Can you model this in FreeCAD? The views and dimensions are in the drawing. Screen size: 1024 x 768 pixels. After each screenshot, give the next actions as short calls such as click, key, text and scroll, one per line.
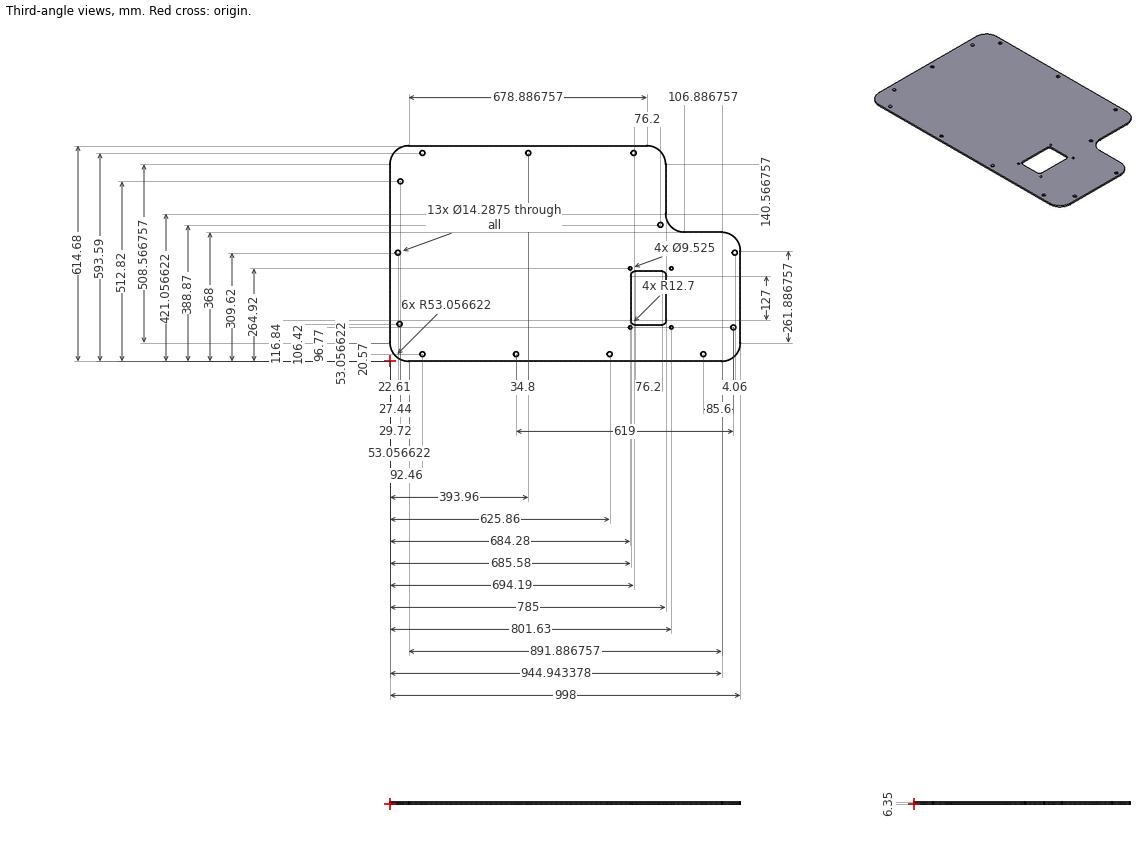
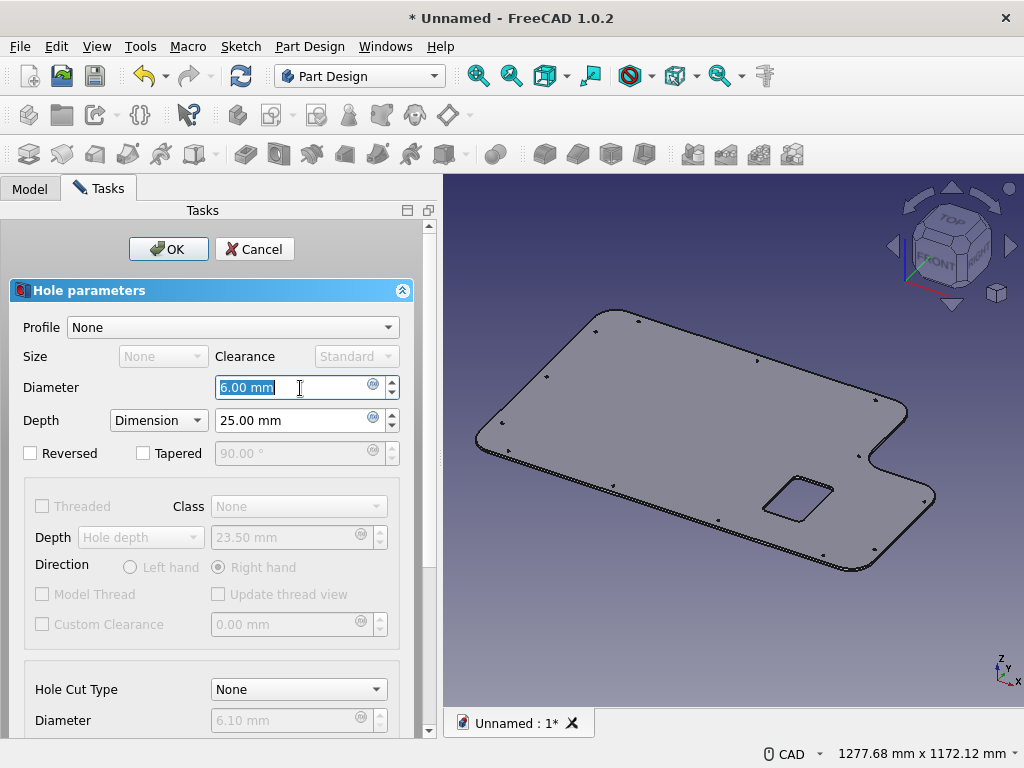
text(14.2875)
key(Tab)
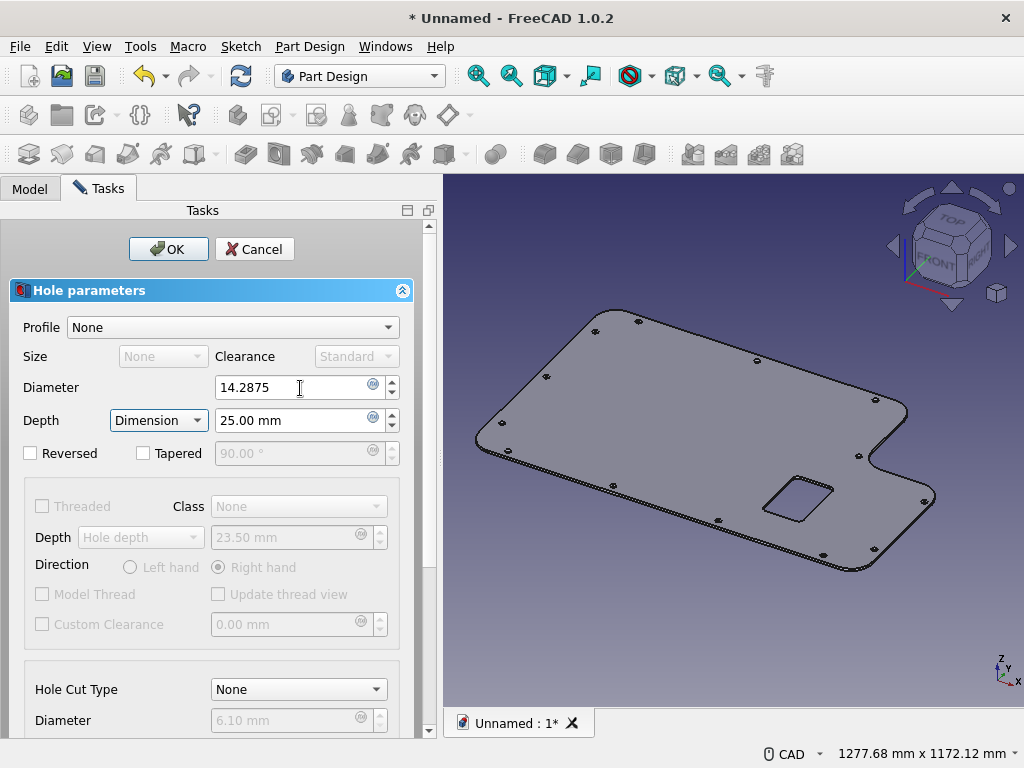
click(160, 420)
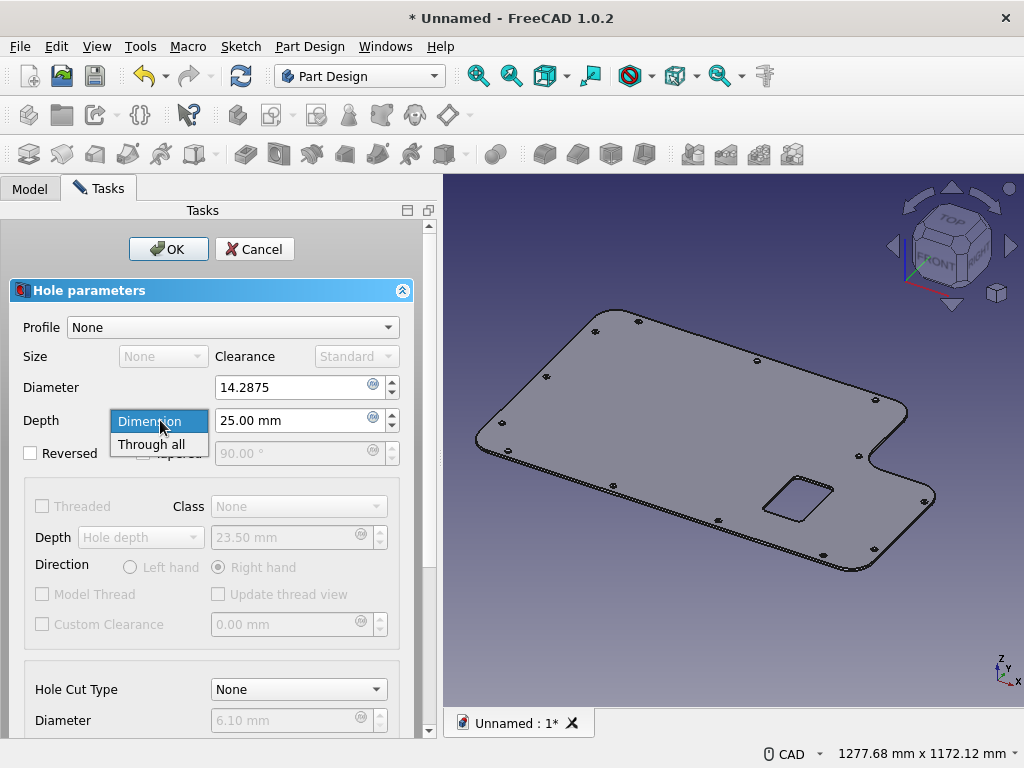
click(158, 444)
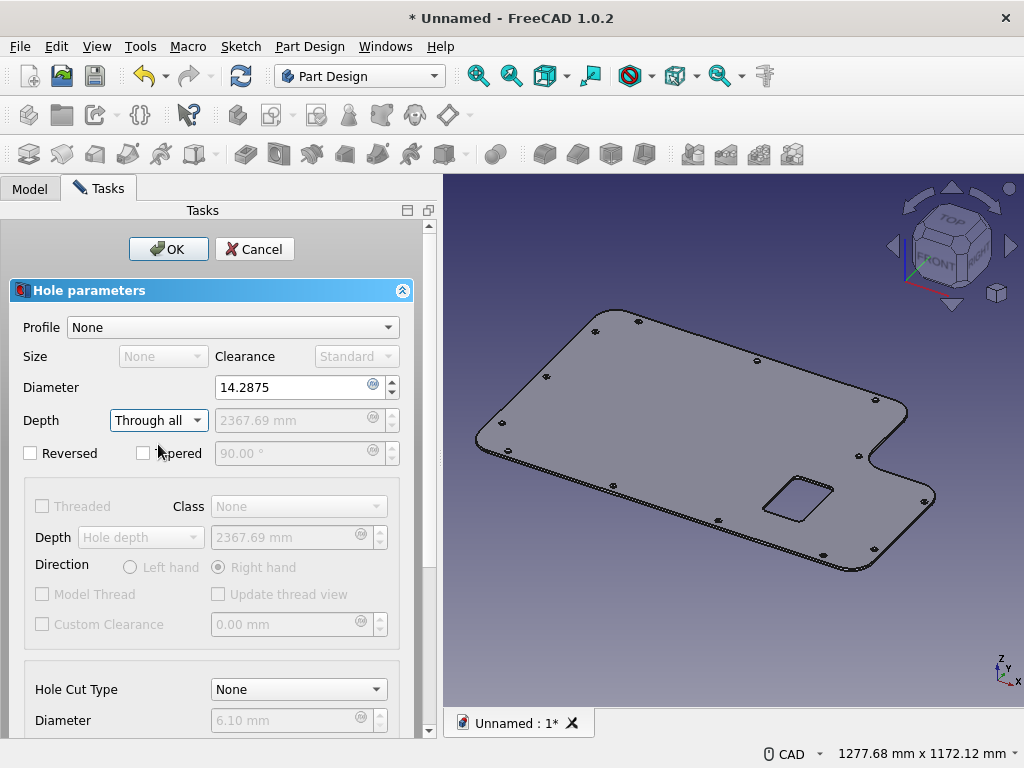
click(169, 249)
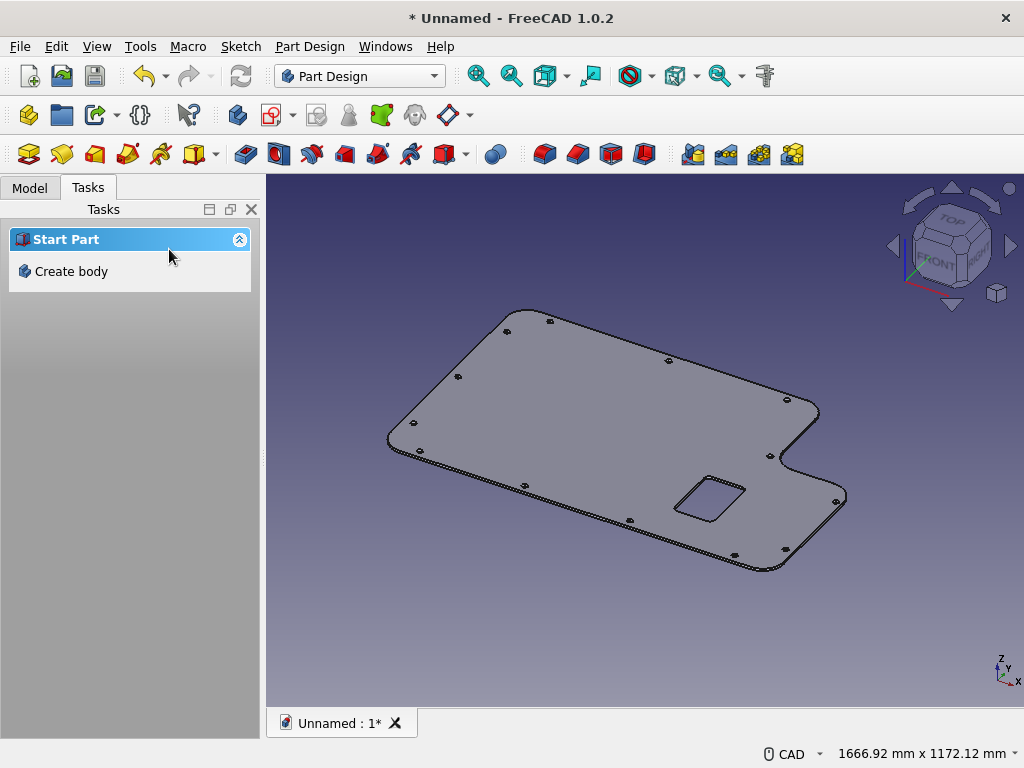
click(589, 420)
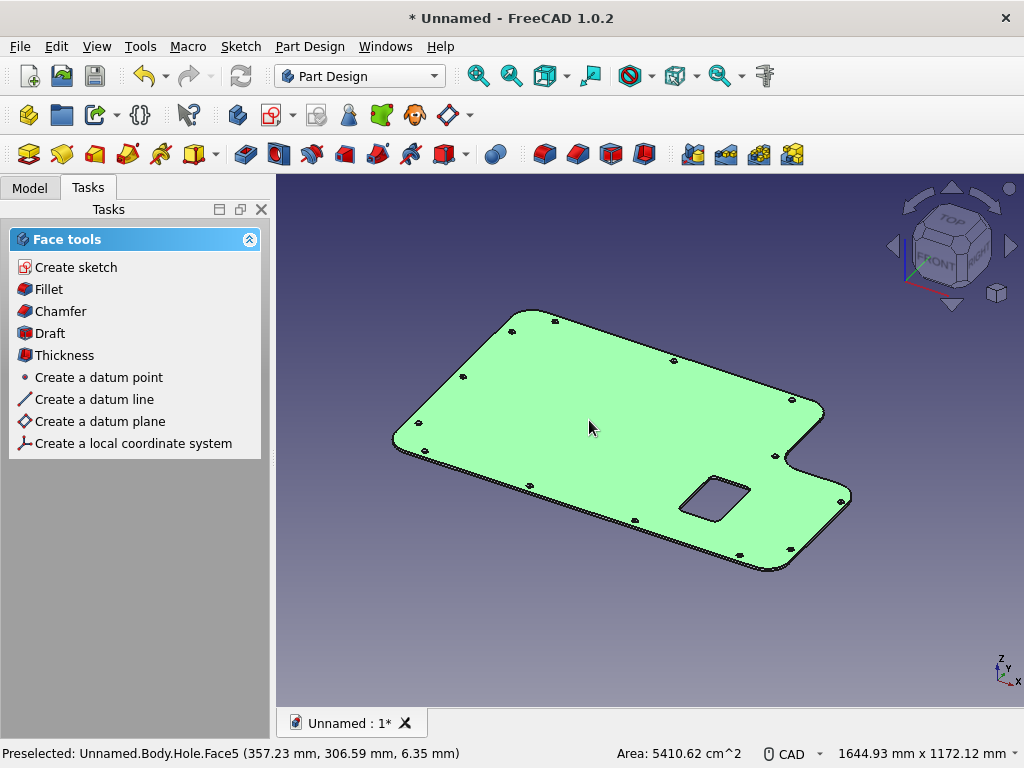
click(270, 116)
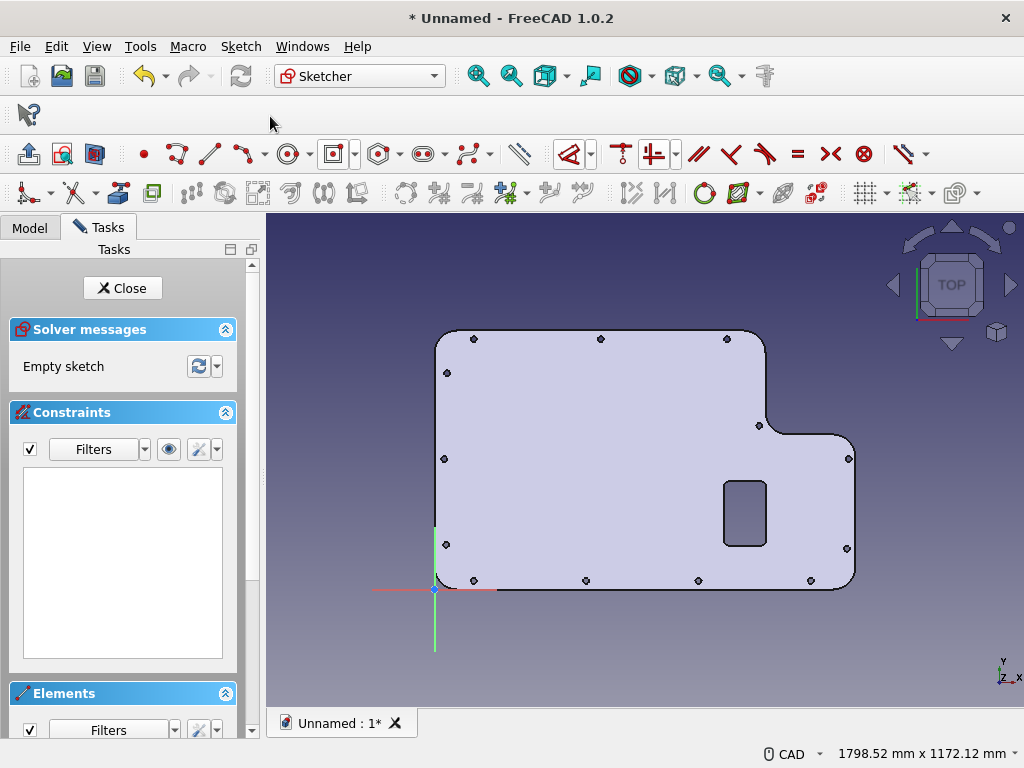
scroll(804, 531, up, 7)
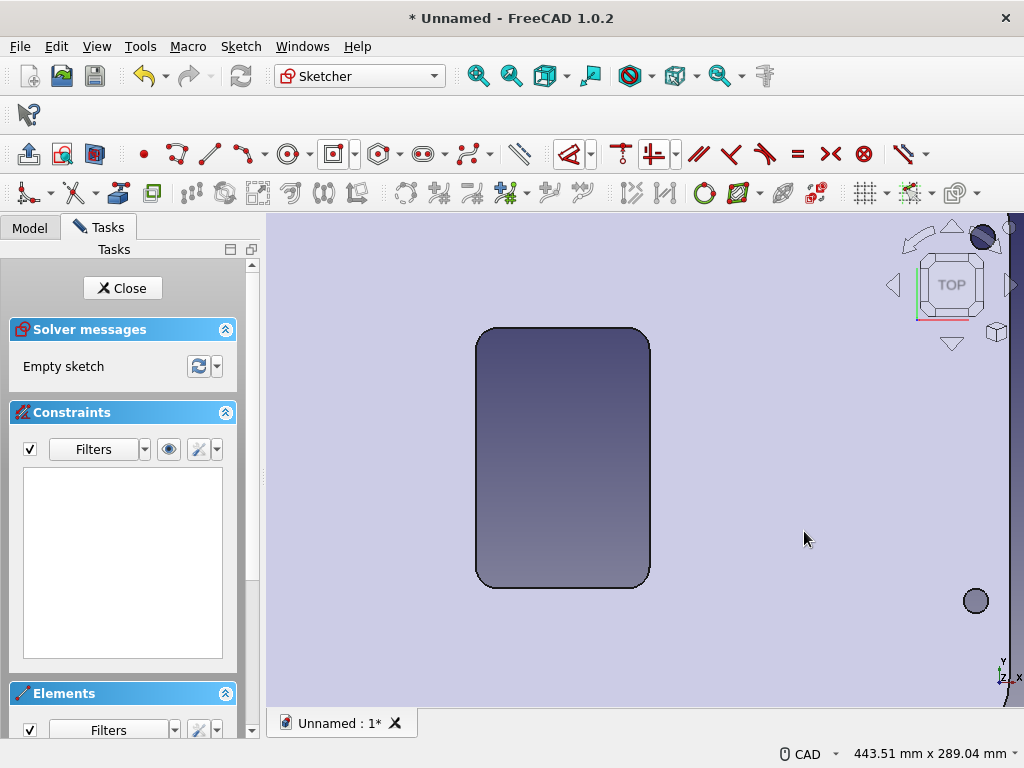
click(288, 154)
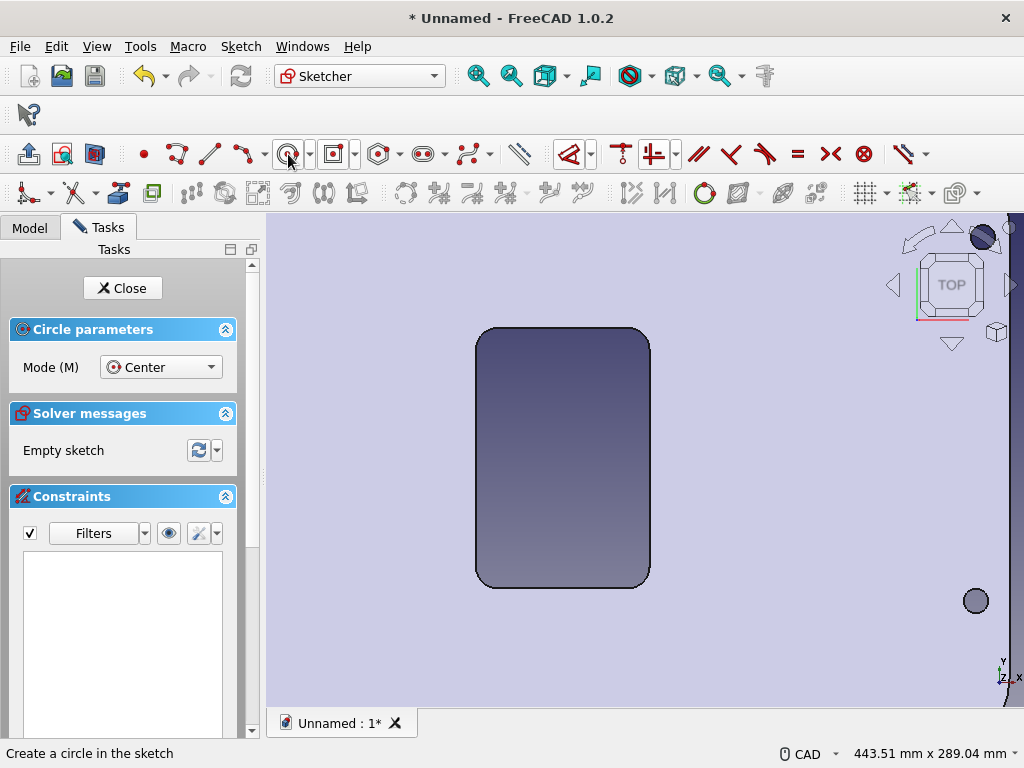
scroll(474, 314, up, 6)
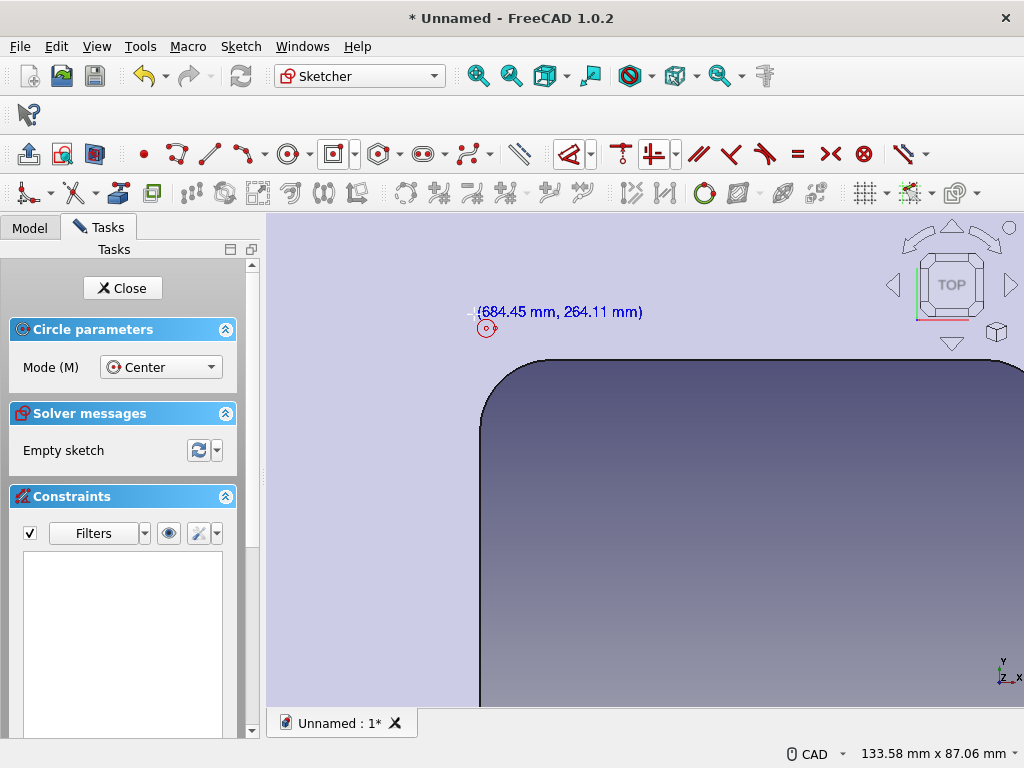
click(472, 312)
move(492, 293)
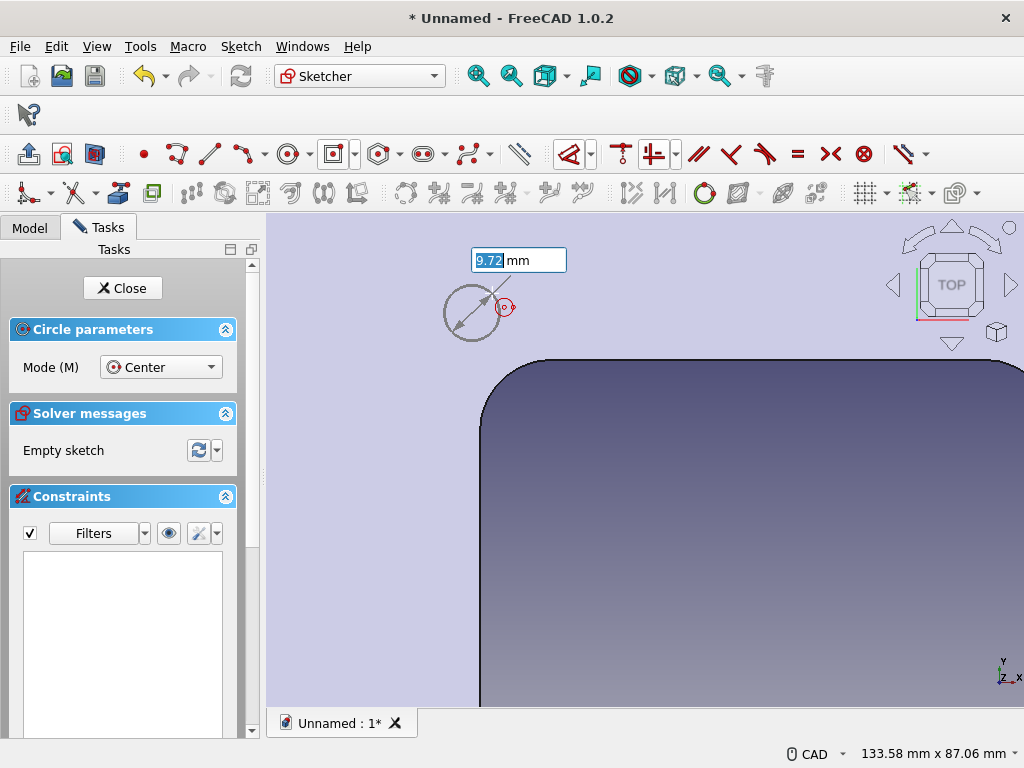
text(9.525)
key(Return)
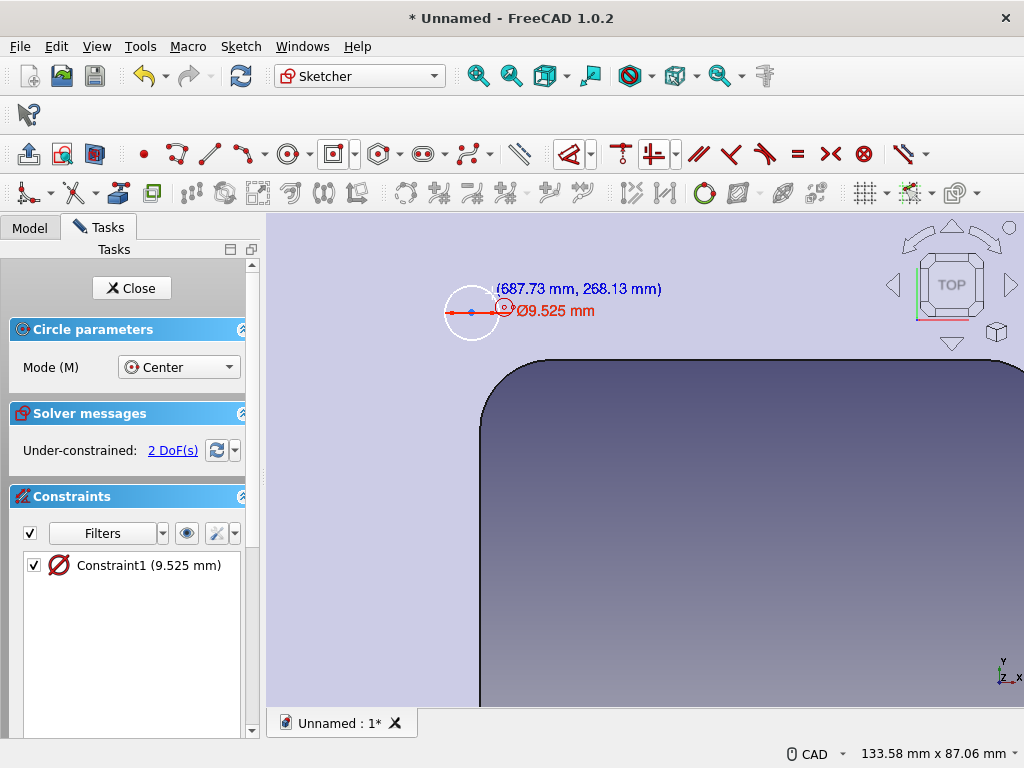
scroll(478, 318, down, 6)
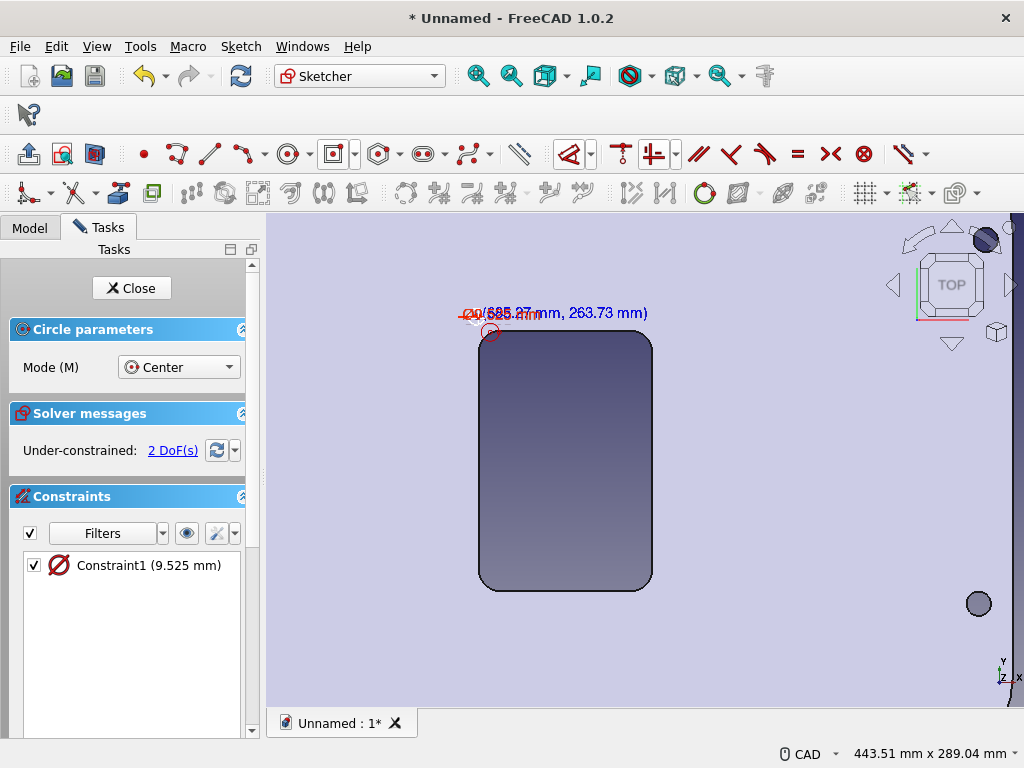
scroll(477, 604, up, 6)